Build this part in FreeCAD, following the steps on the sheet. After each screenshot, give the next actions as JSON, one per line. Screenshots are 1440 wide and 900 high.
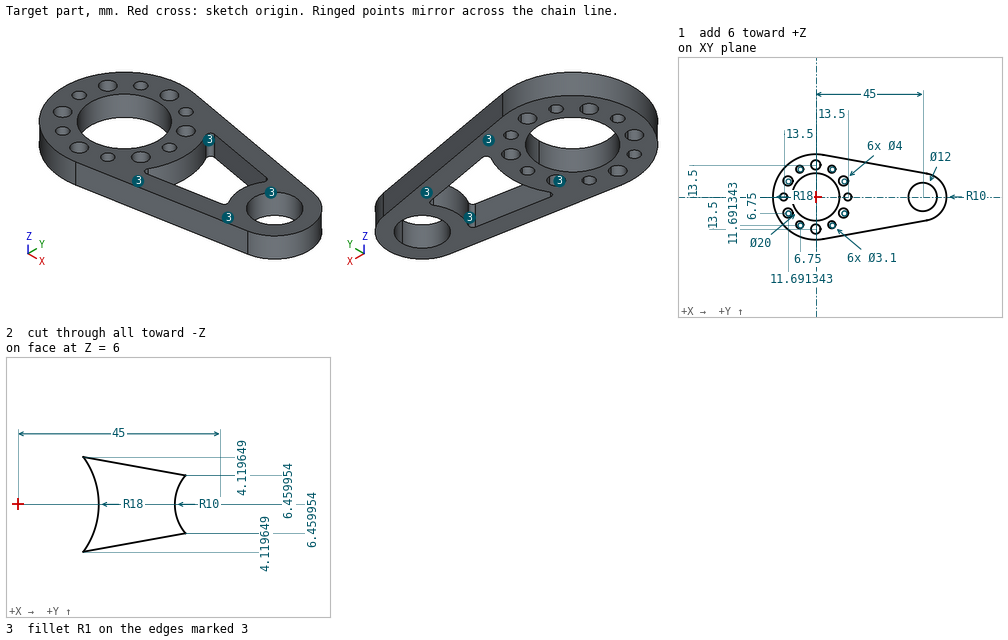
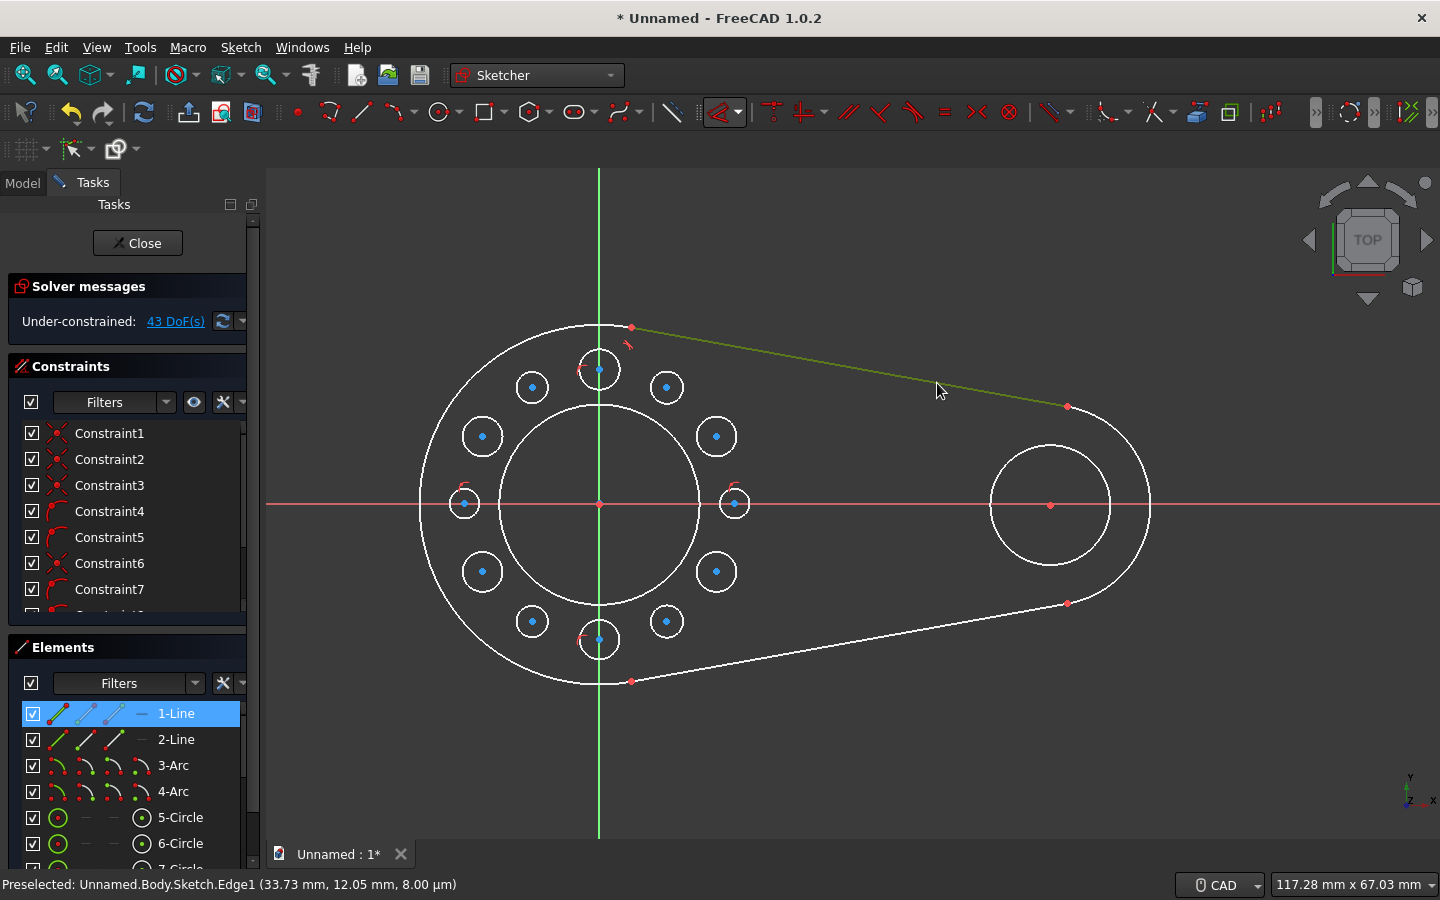
{"action": "left_click", "coordinate": [1135, 558]}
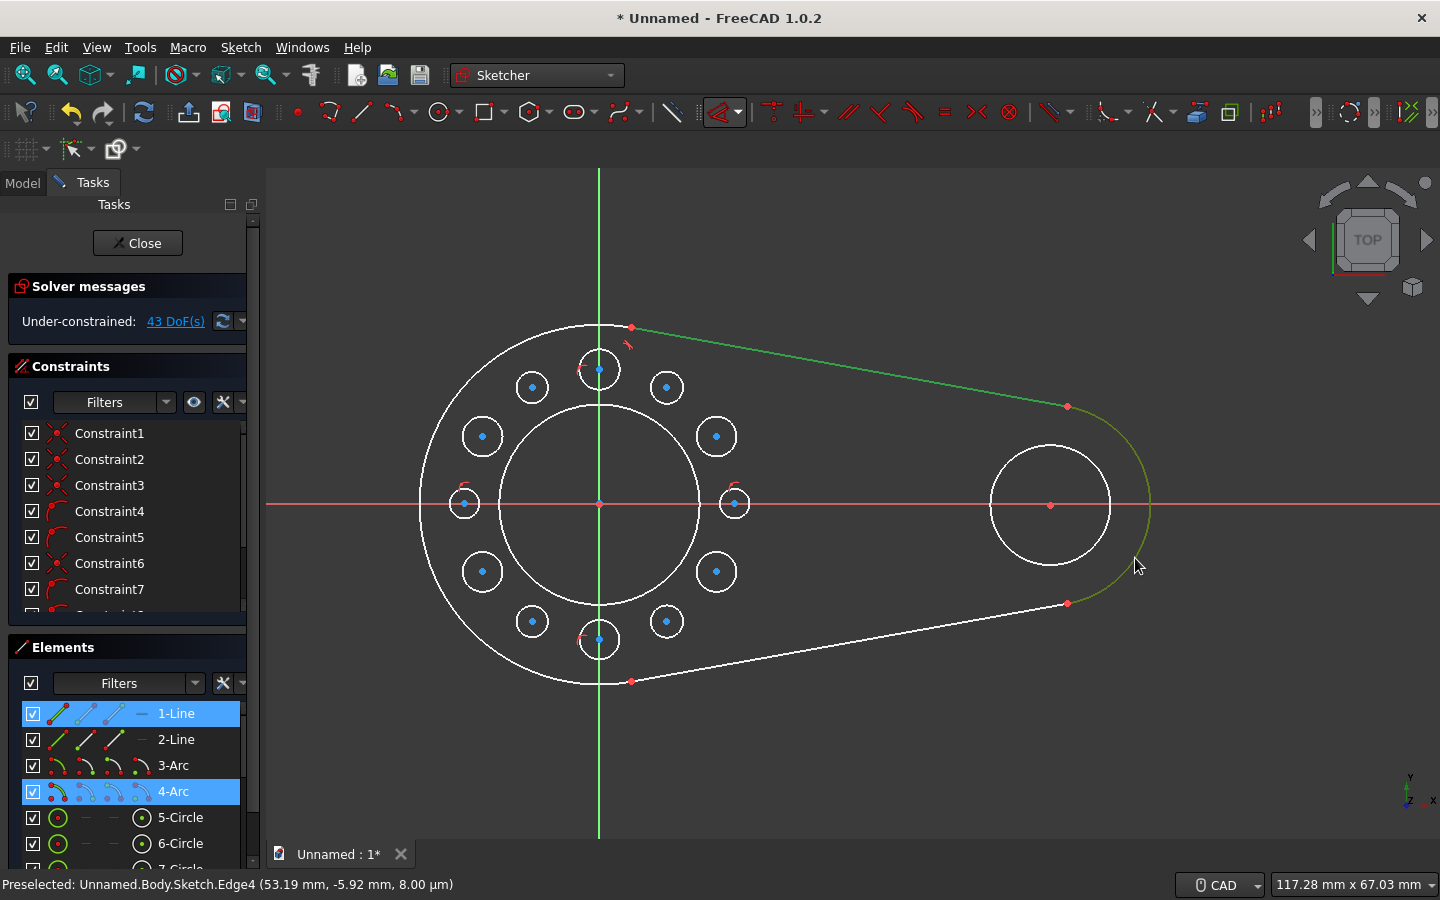
{"action": "left_click", "coordinate": [914, 112]}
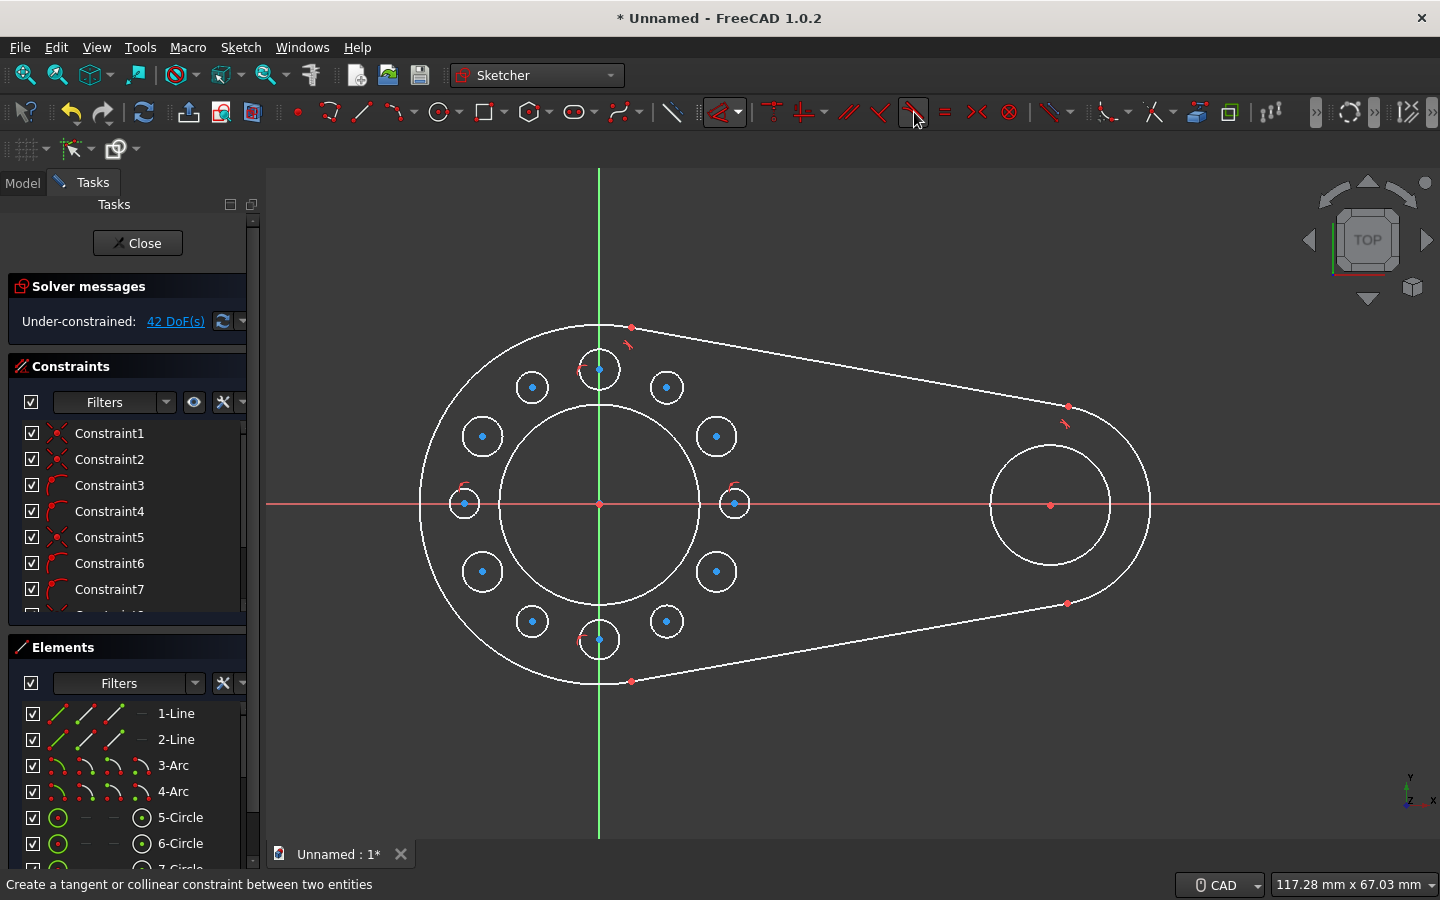
{"action": "left_click", "coordinate": [762, 658]}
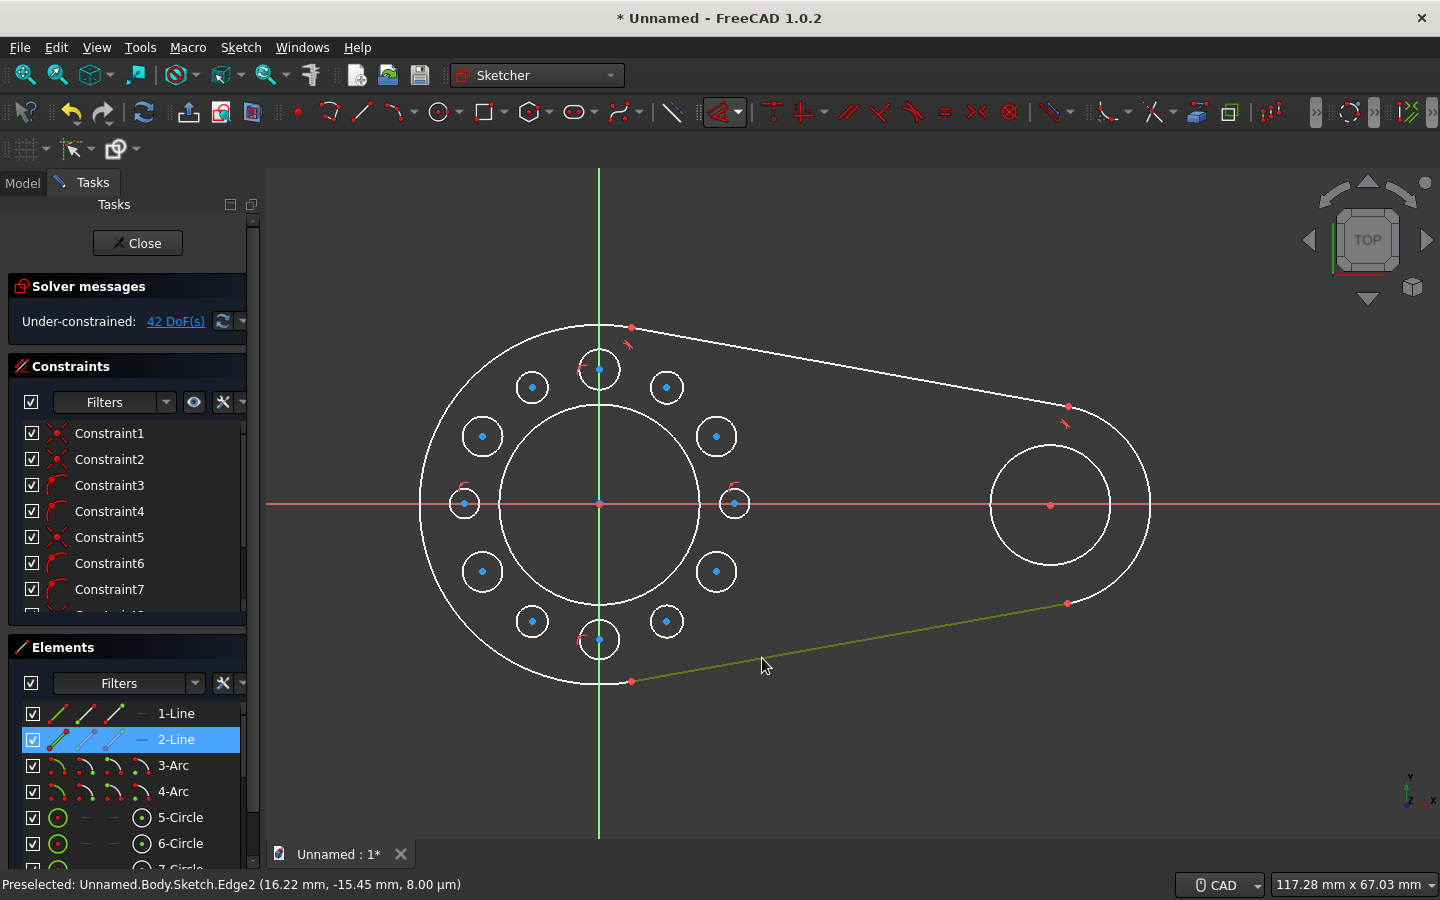
{"action": "left_click", "coordinate": [462, 389]}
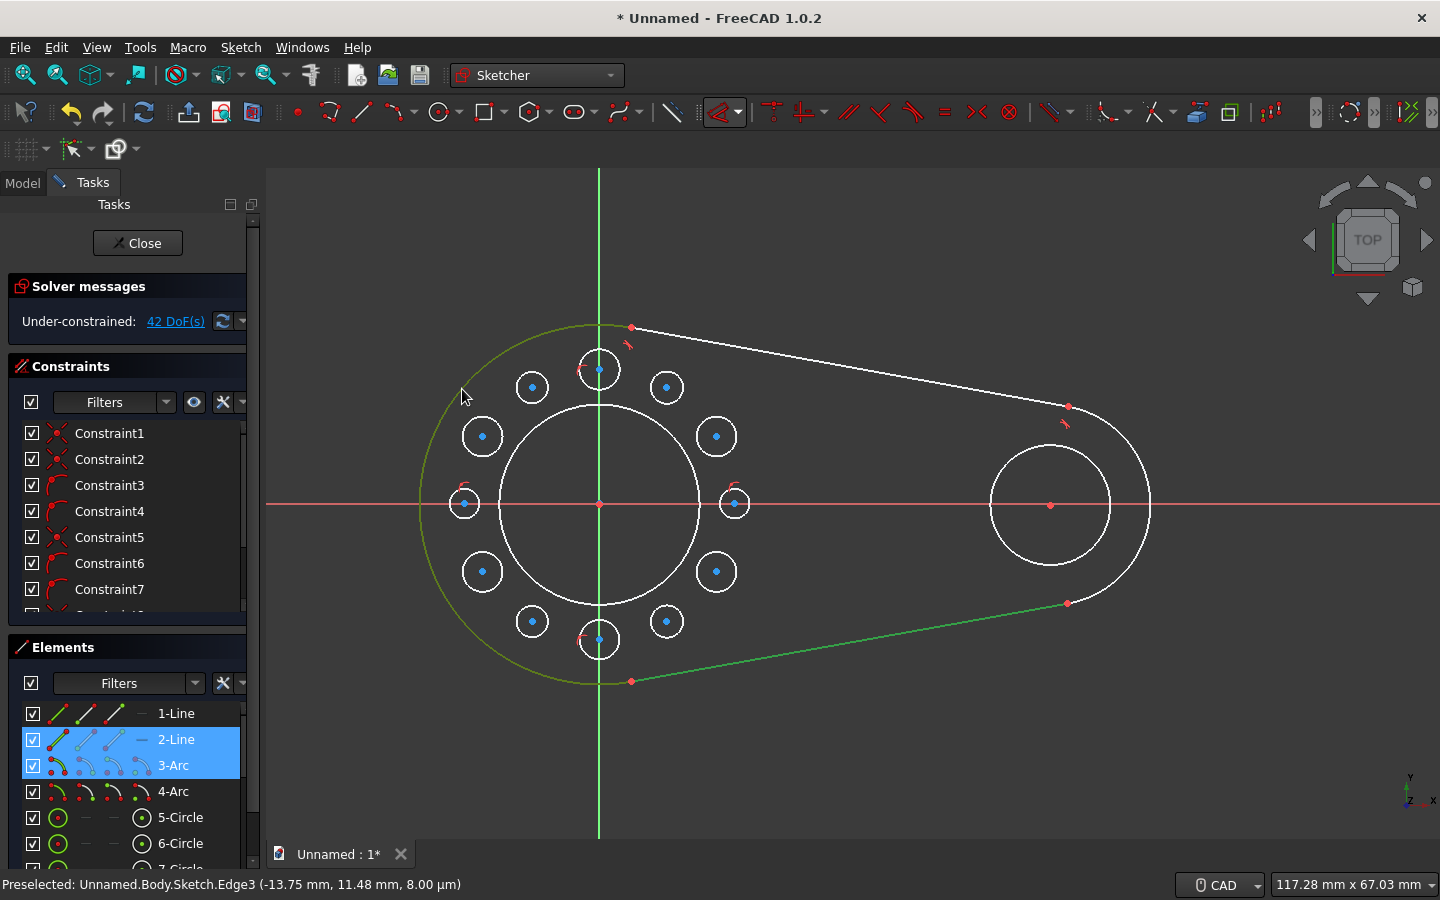
{"action": "key", "text": "t"}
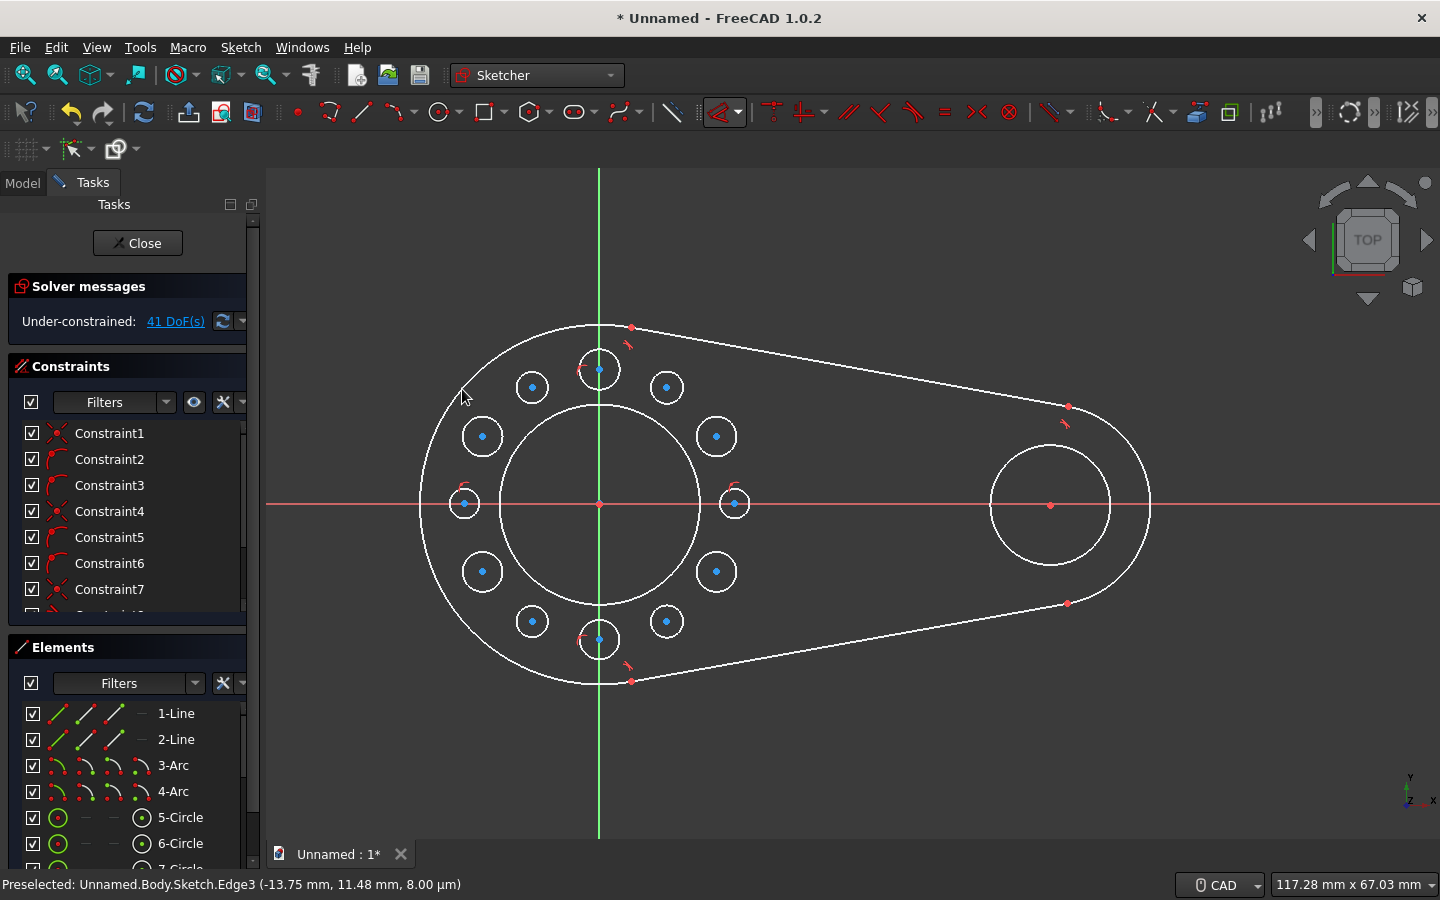
{"action": "left_click", "coordinate": [762, 658]}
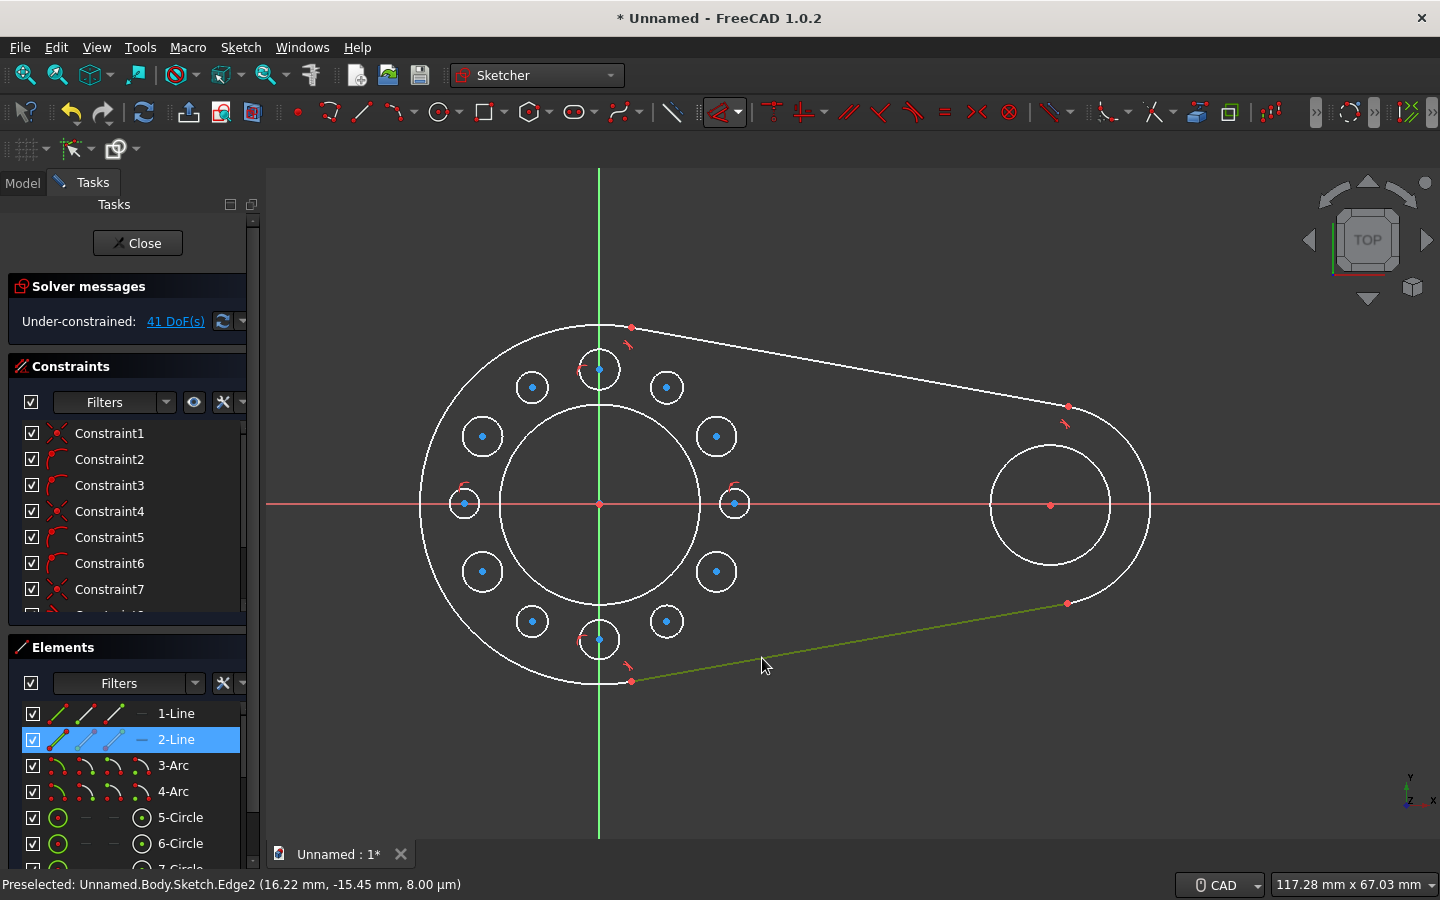
{"action": "left_click", "coordinate": [1135, 558]}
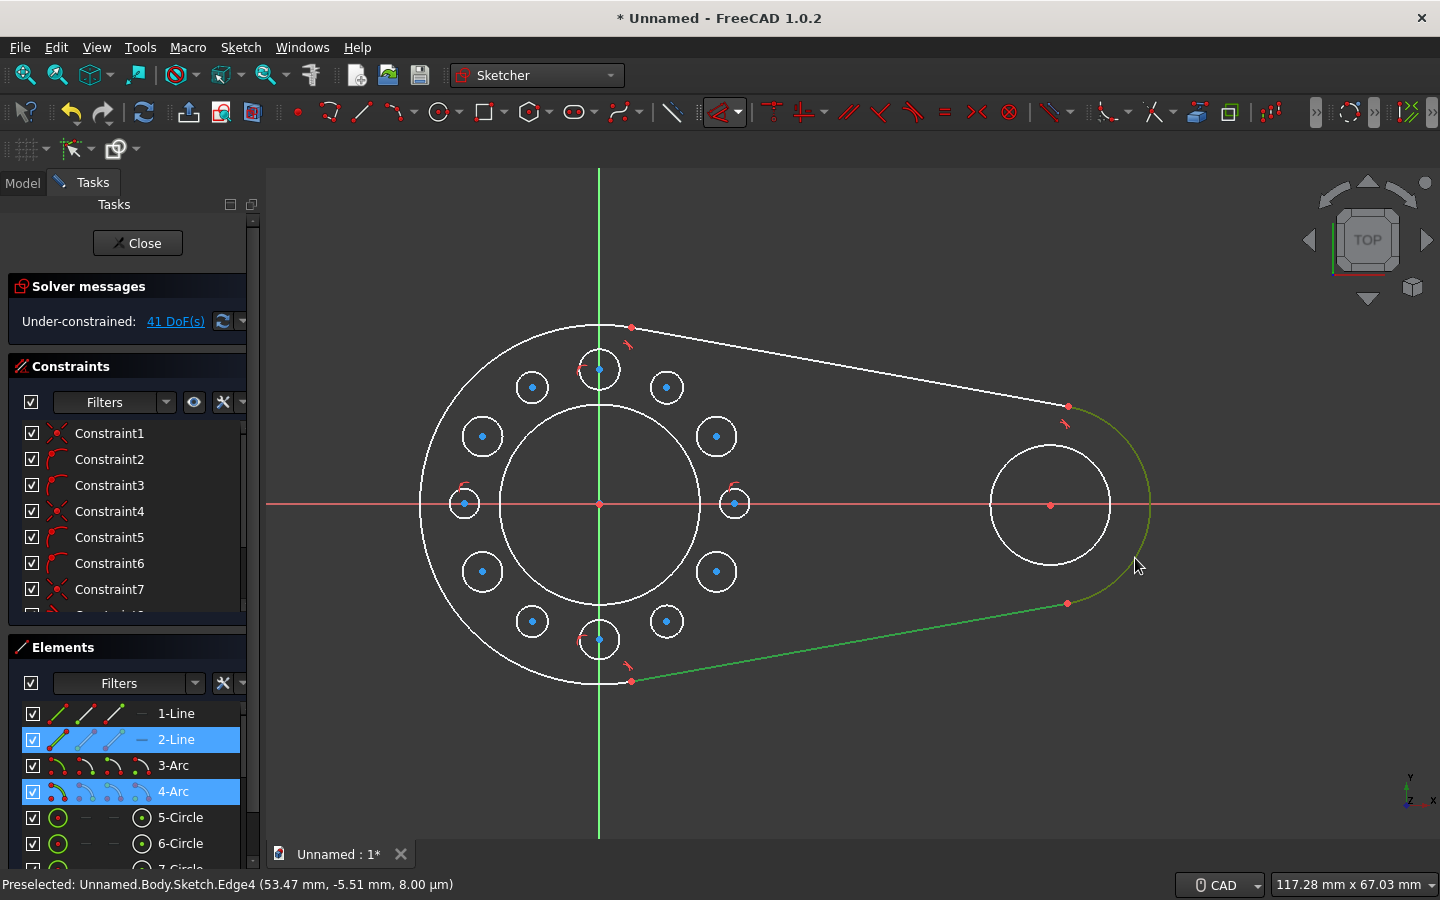
{"action": "left_click", "coordinate": [914, 112]}